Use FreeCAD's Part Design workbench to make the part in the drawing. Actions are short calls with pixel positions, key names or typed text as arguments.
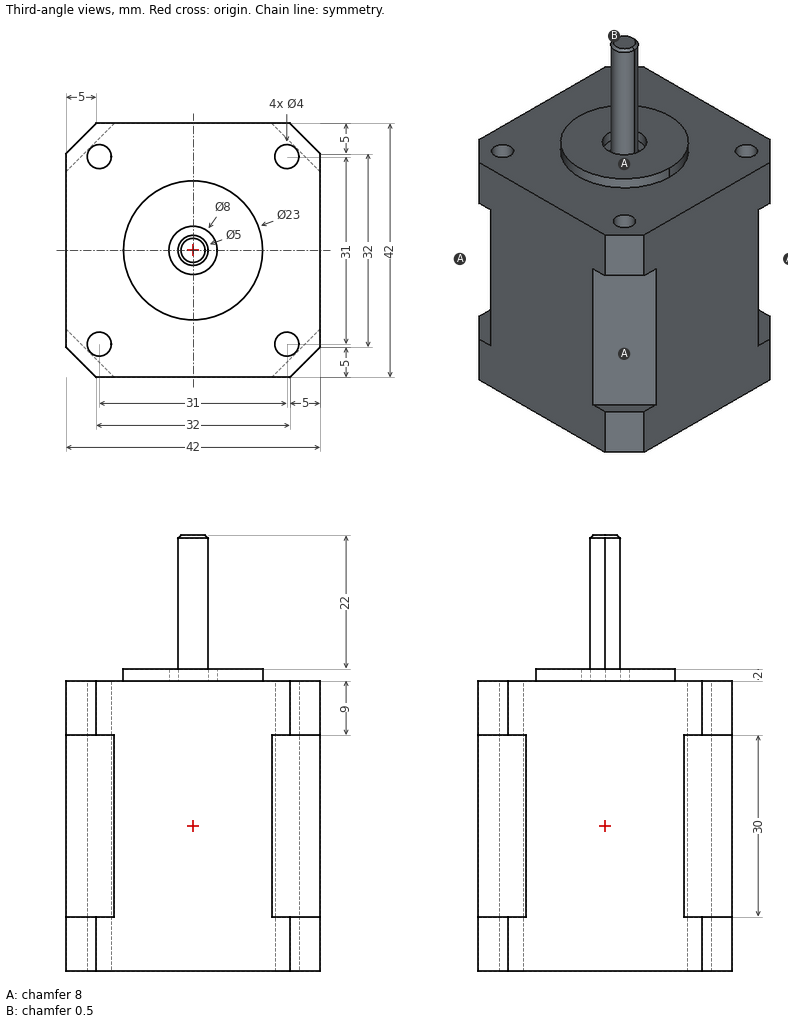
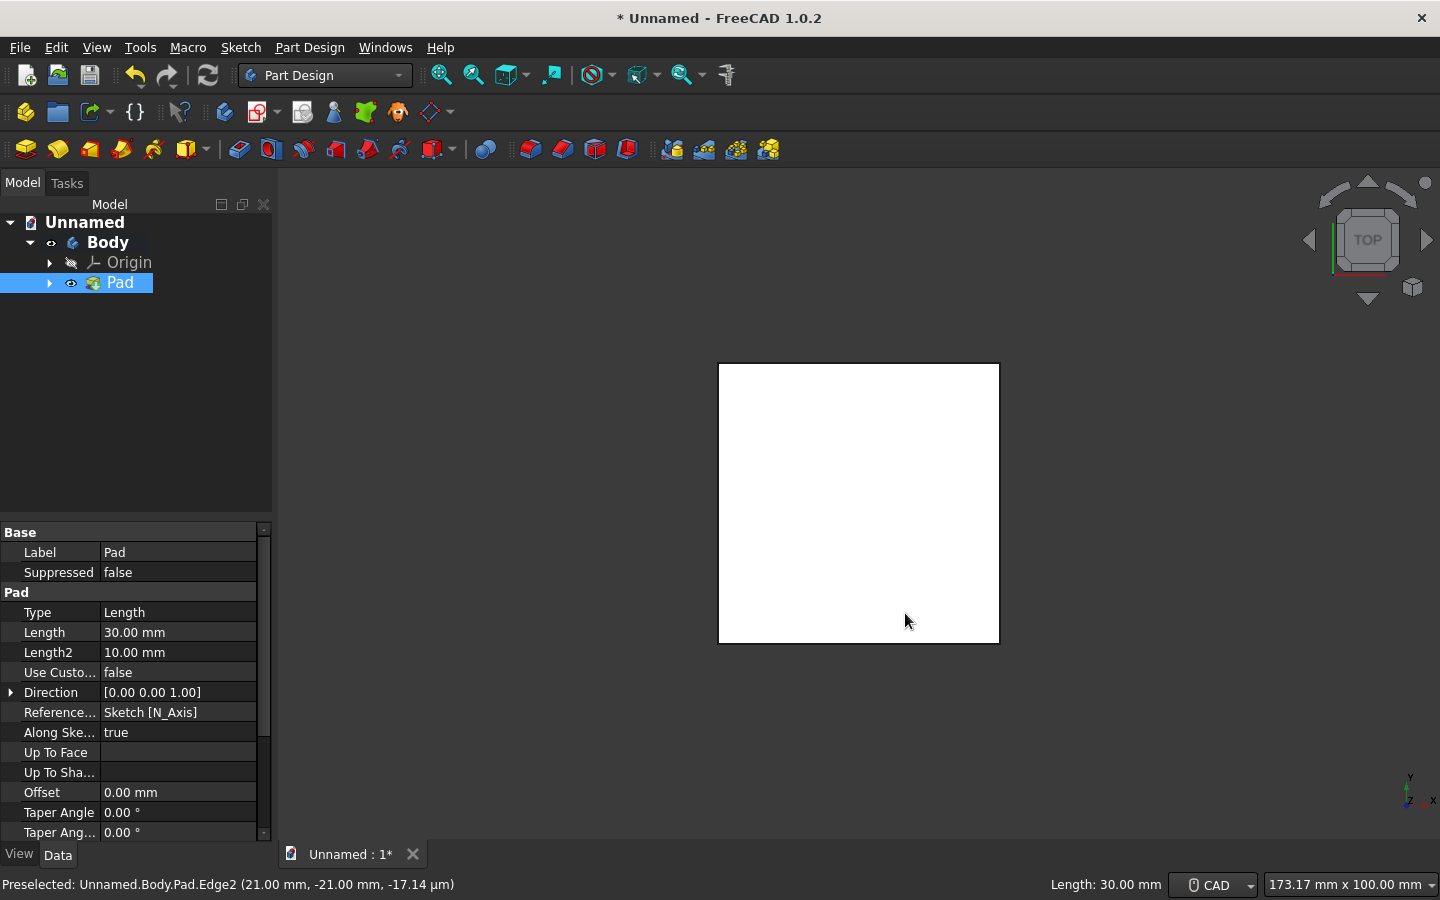
click(442, 76)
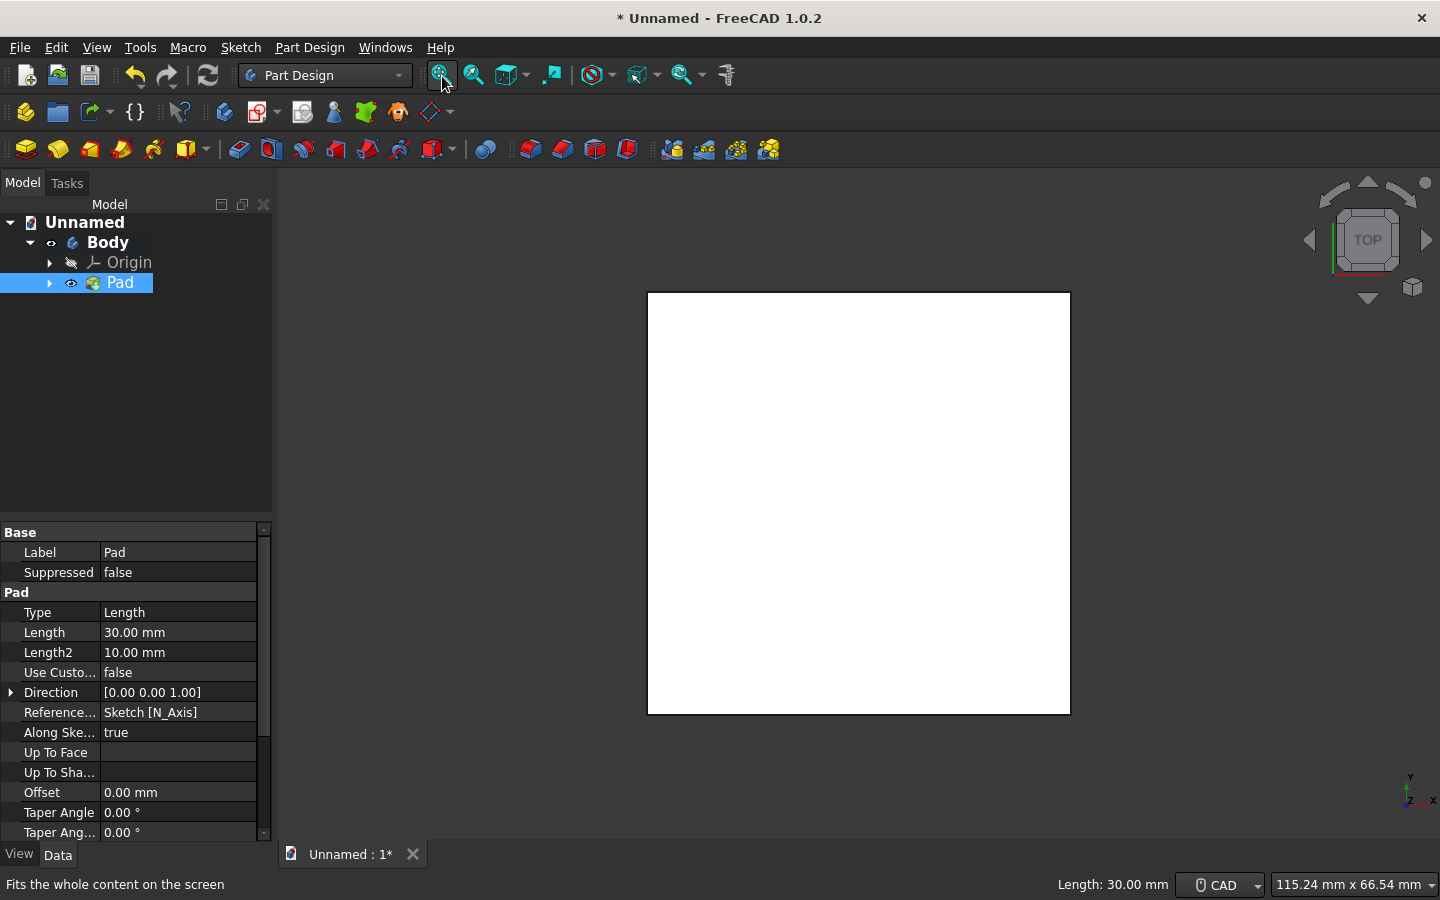
key(1)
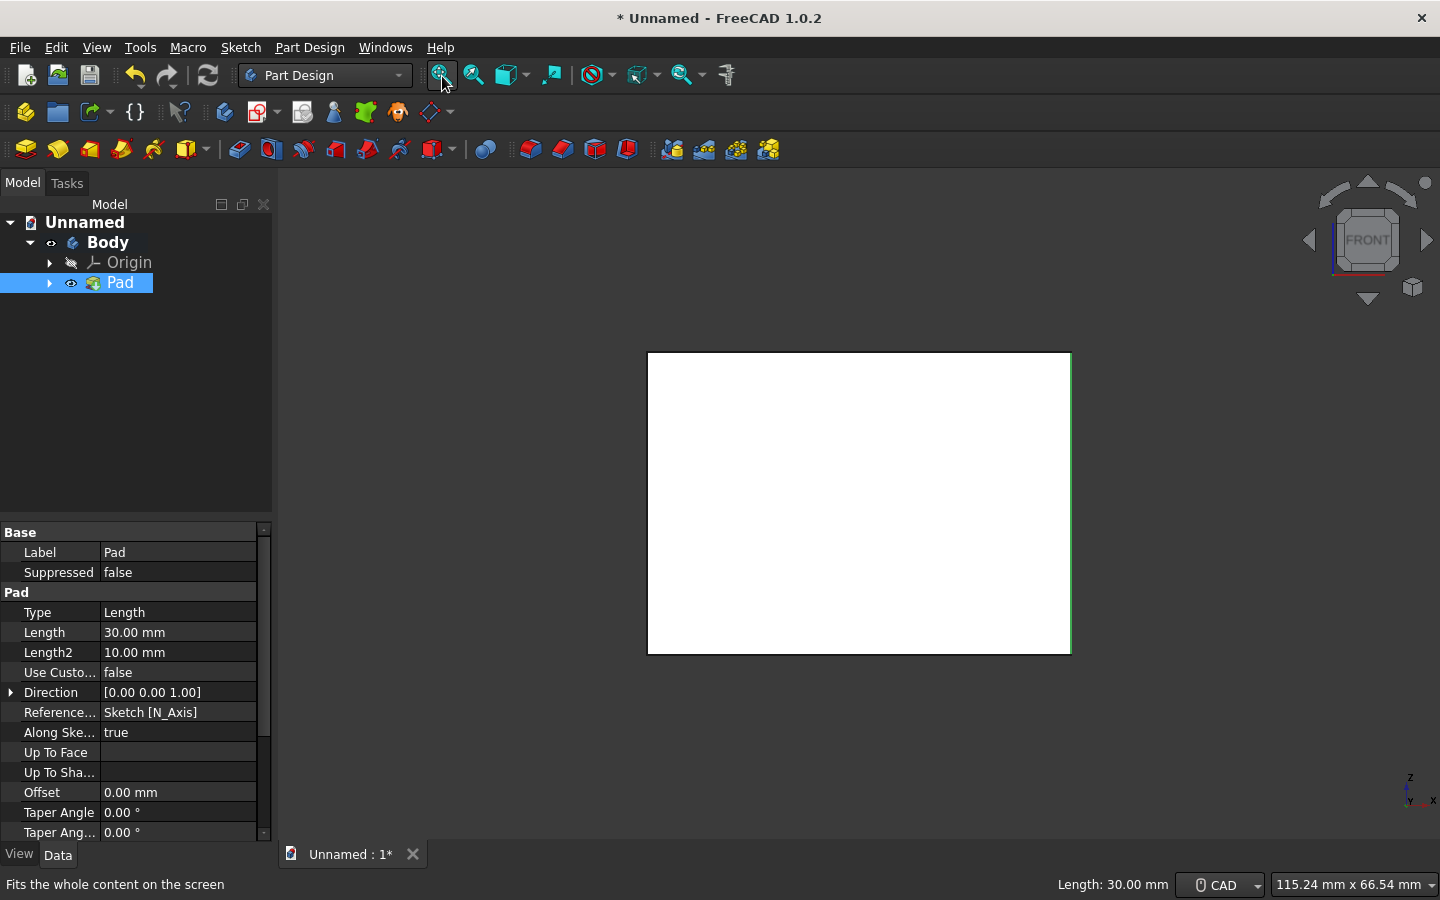
click(647, 502, ctrl)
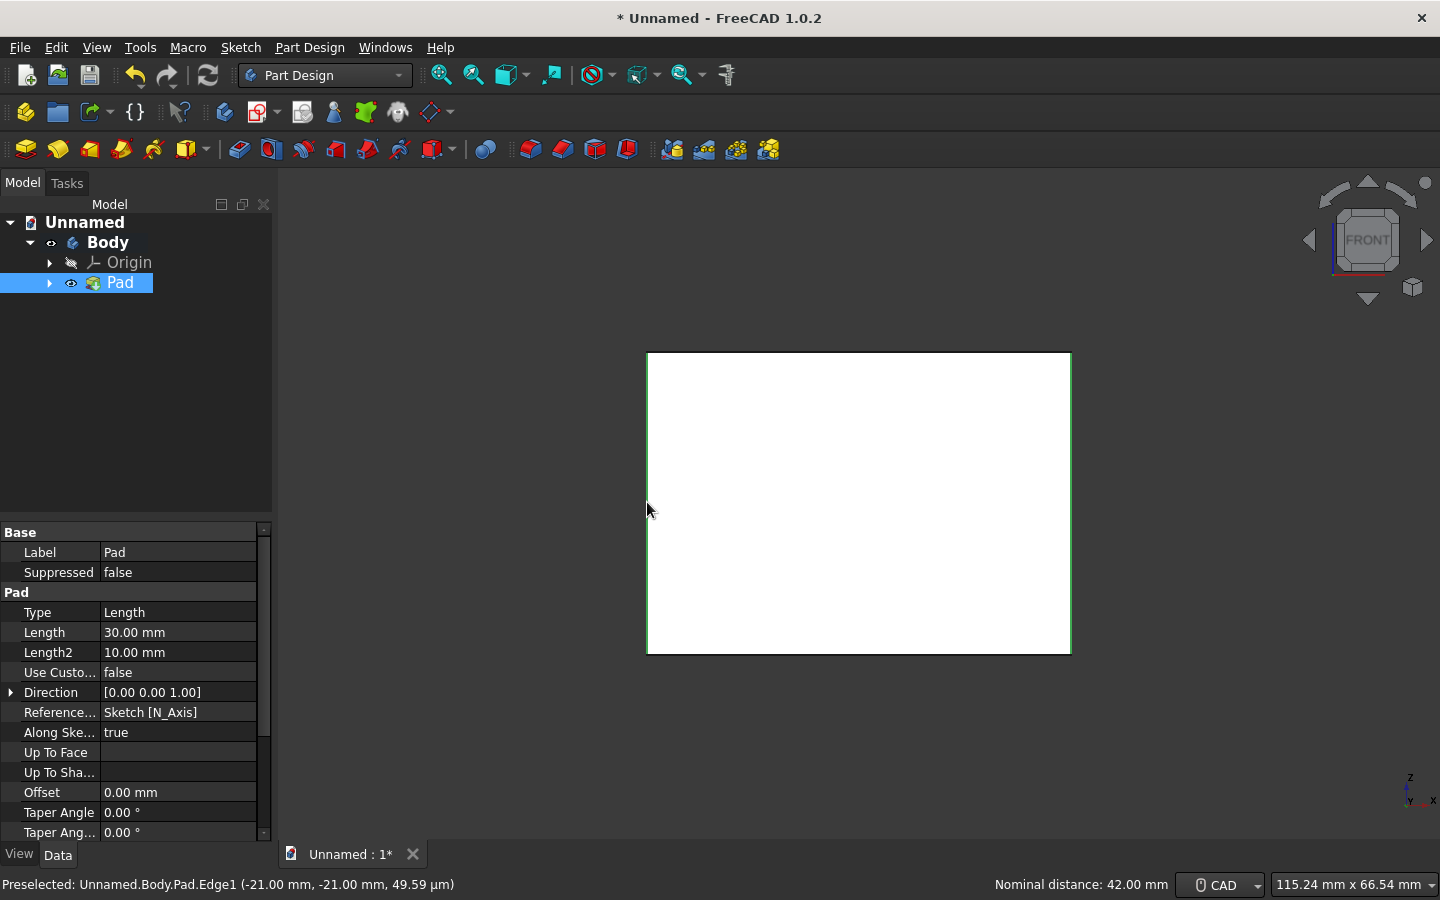
key(3)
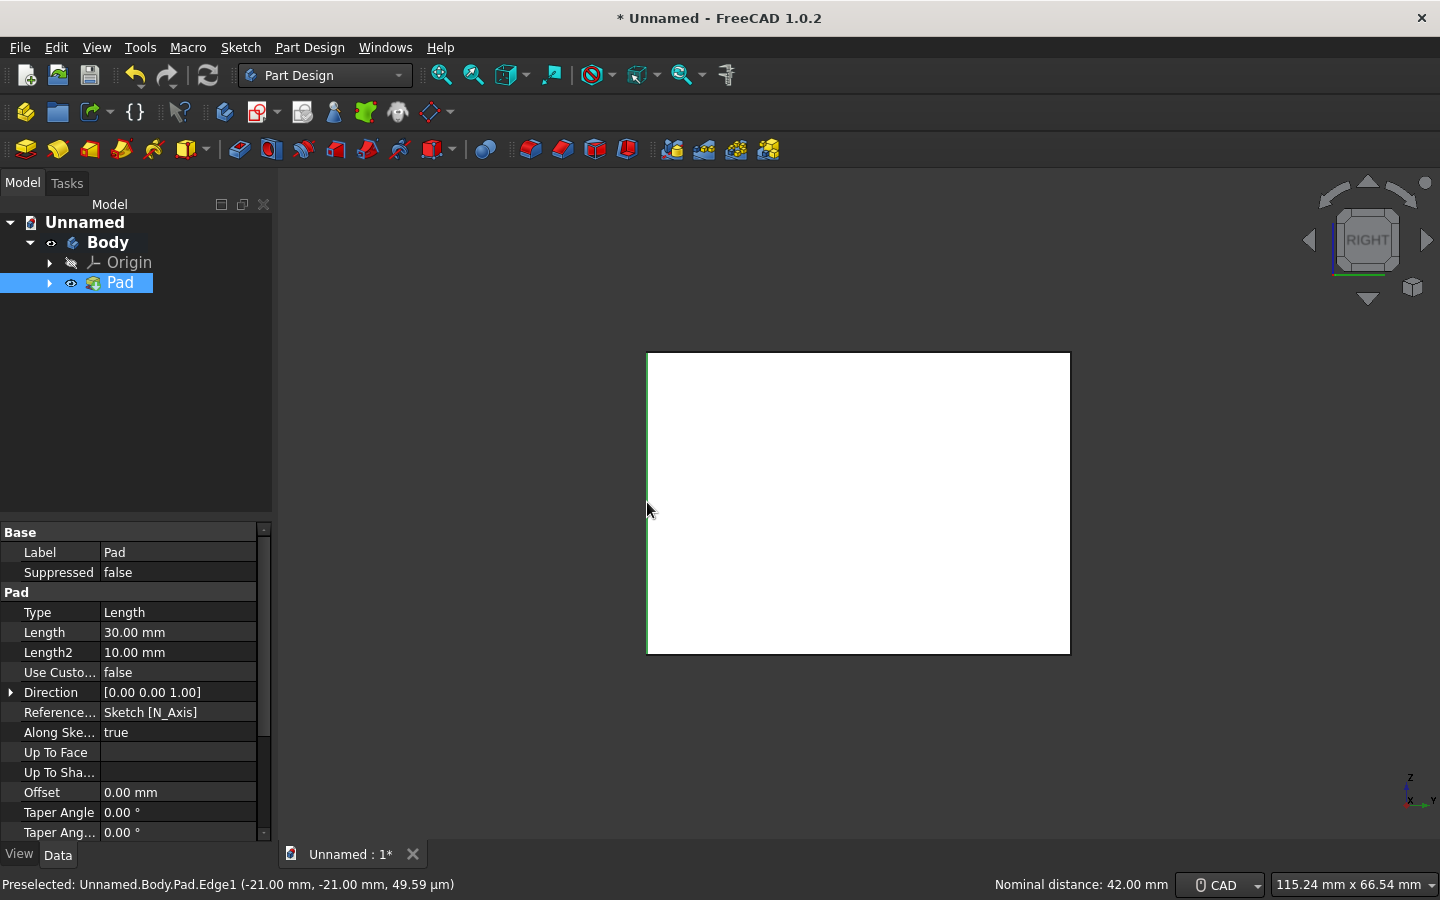
click(1071, 502, ctrl)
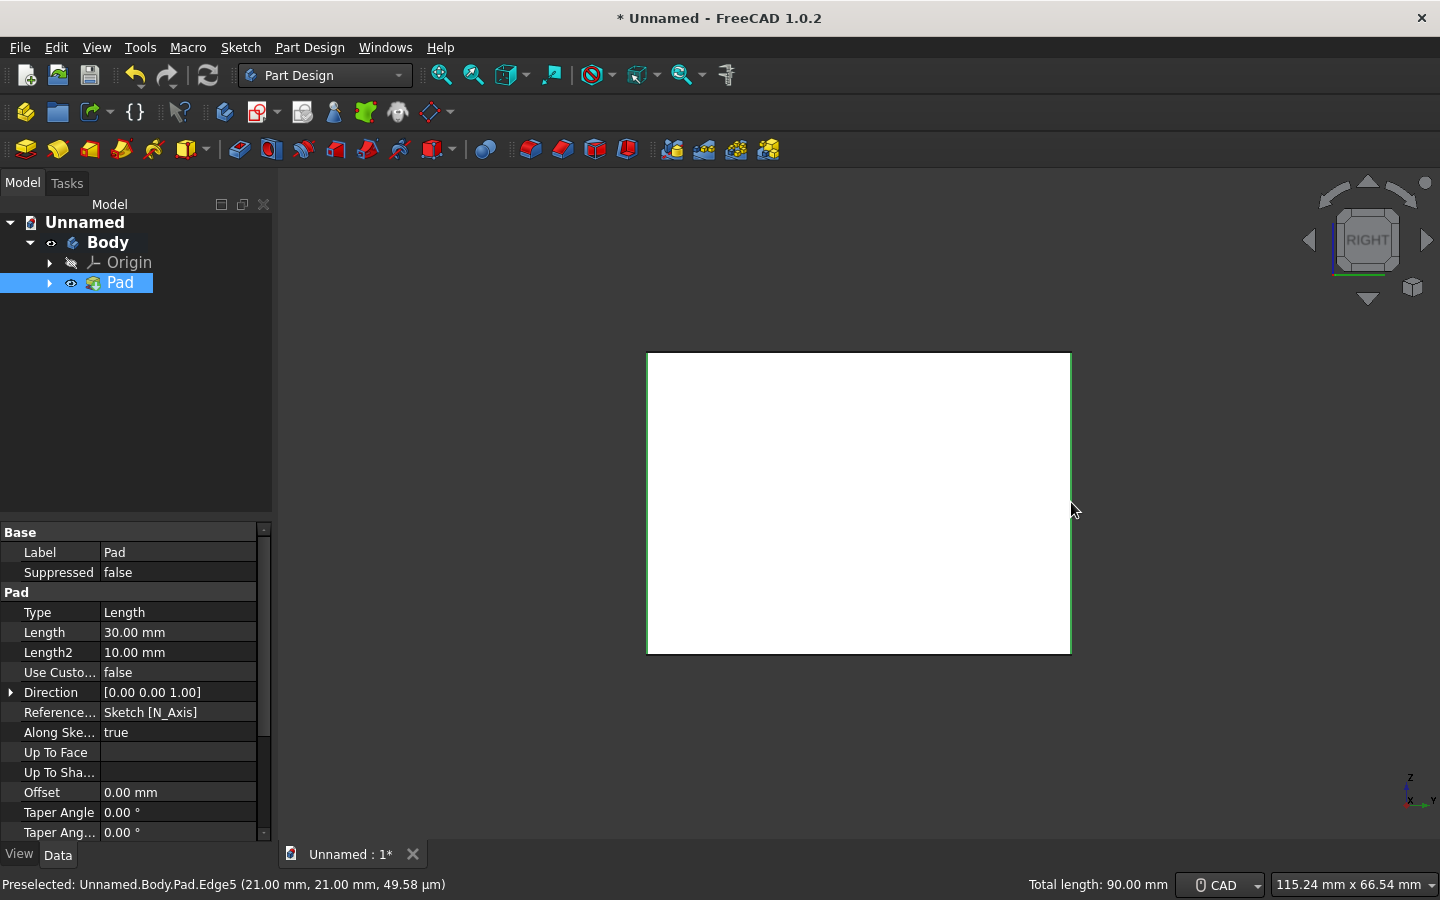
key(5)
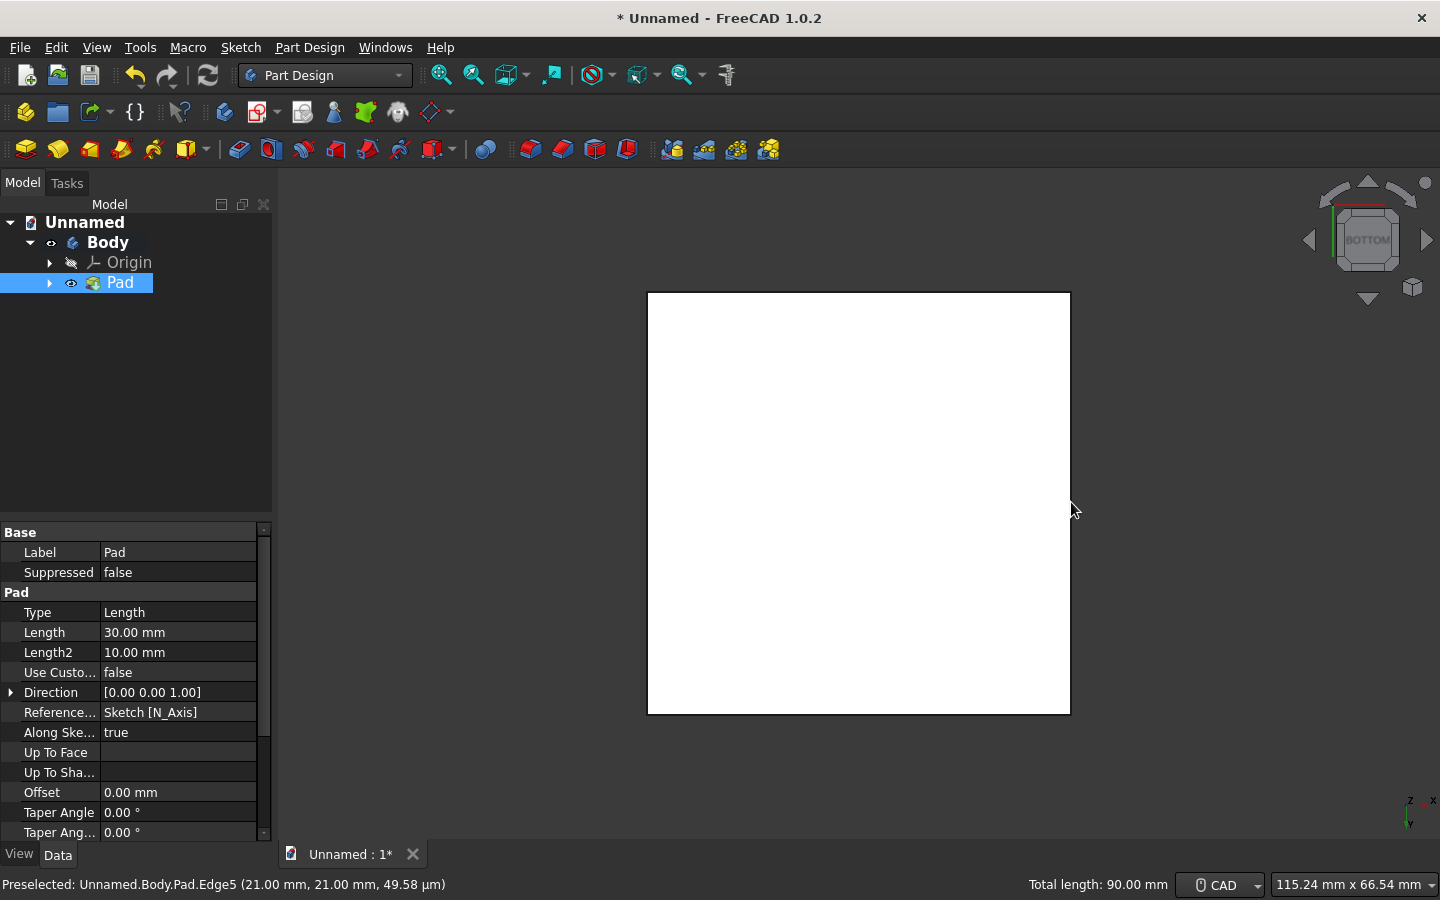
key(4)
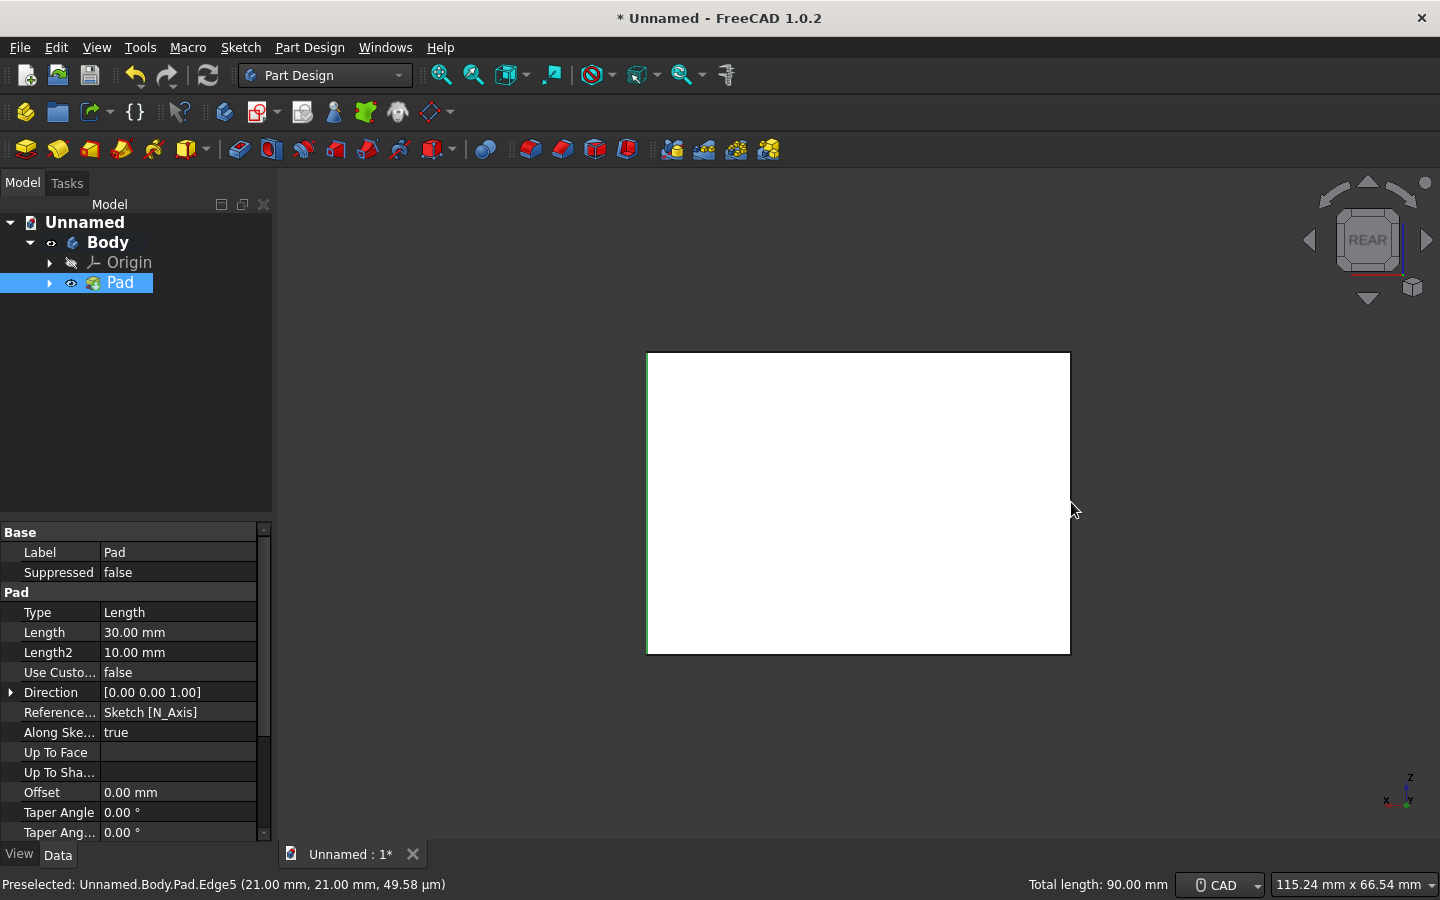
click(1071, 502, ctrl)